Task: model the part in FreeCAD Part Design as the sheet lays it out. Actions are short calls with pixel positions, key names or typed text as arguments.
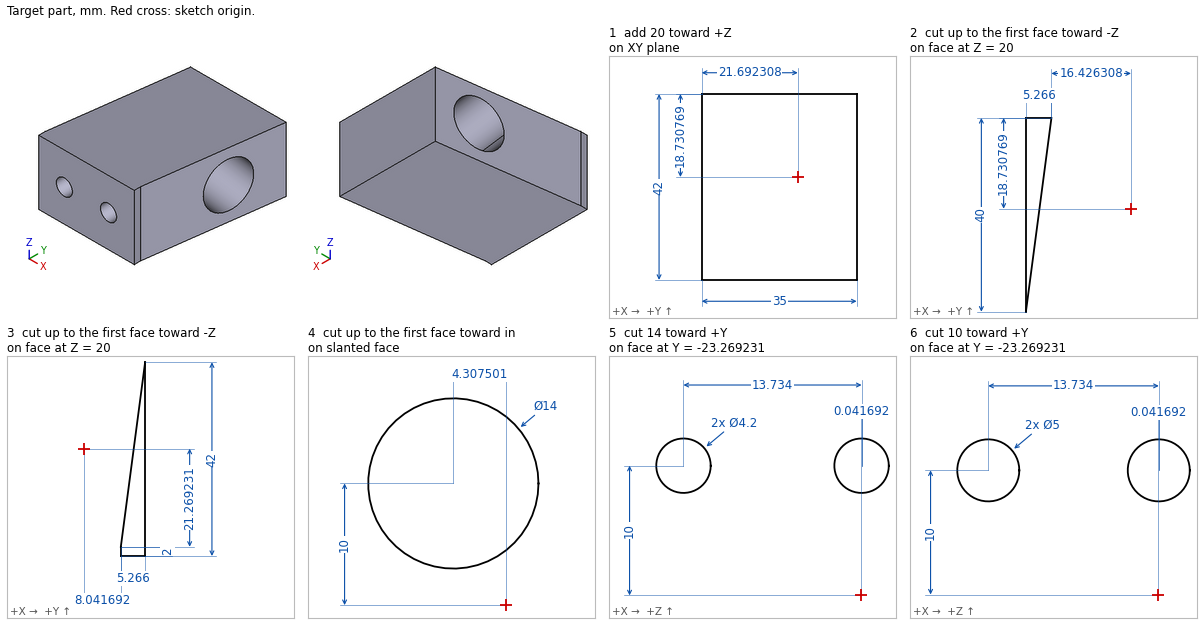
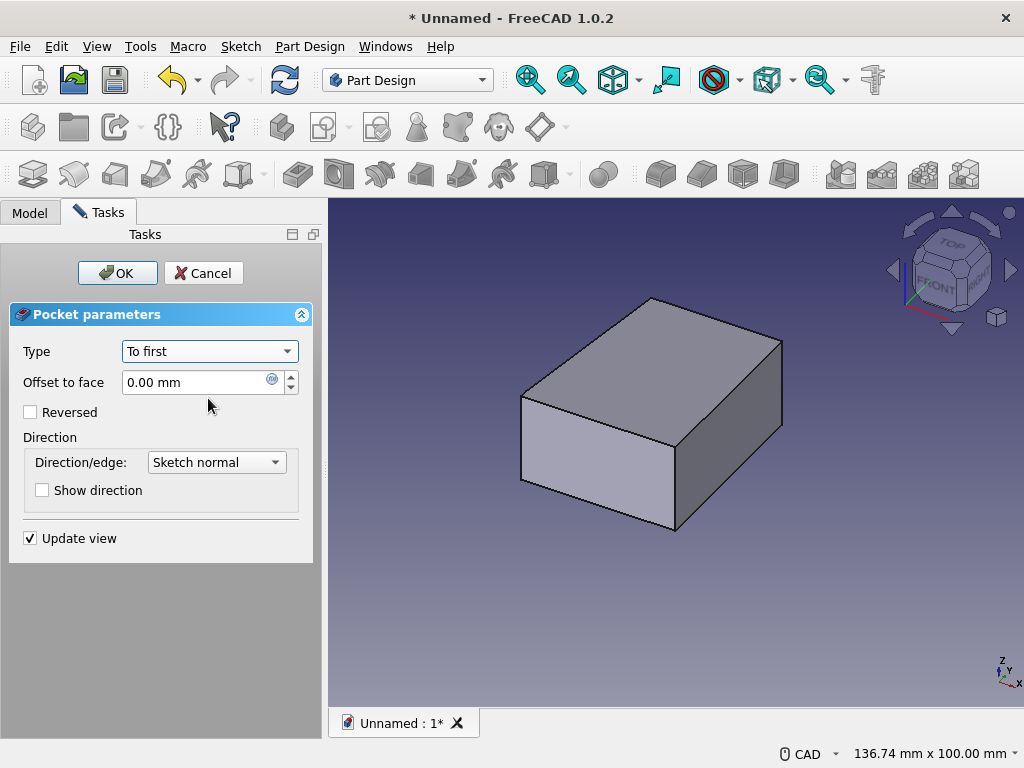
click(118, 273)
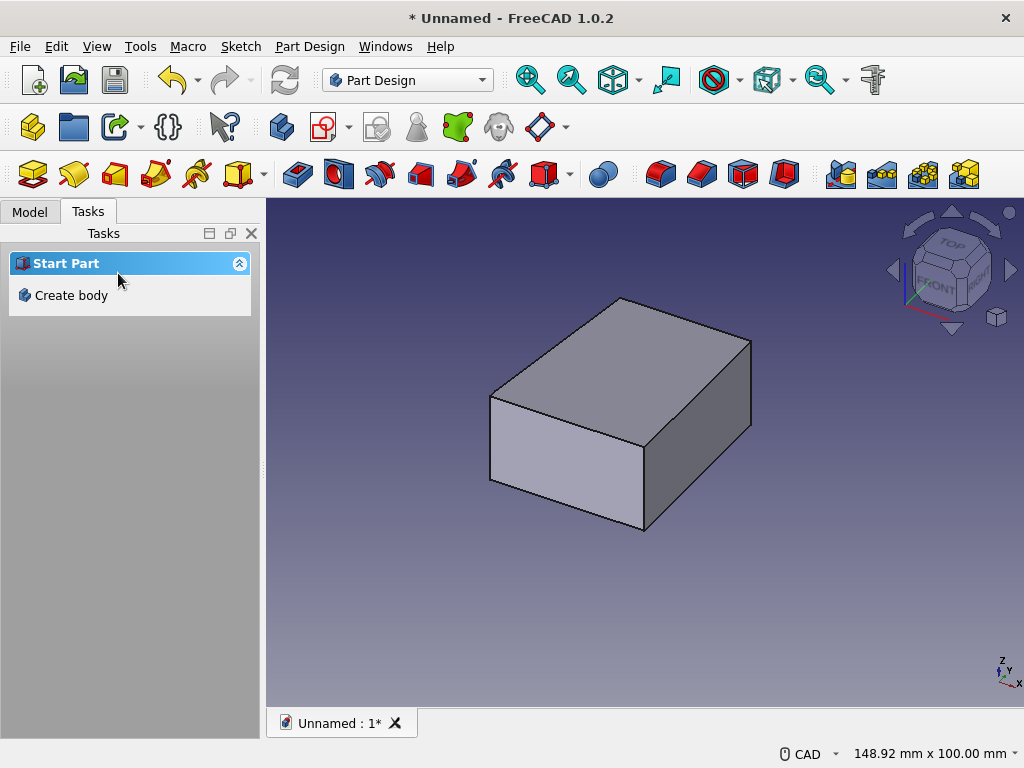
click(605, 383)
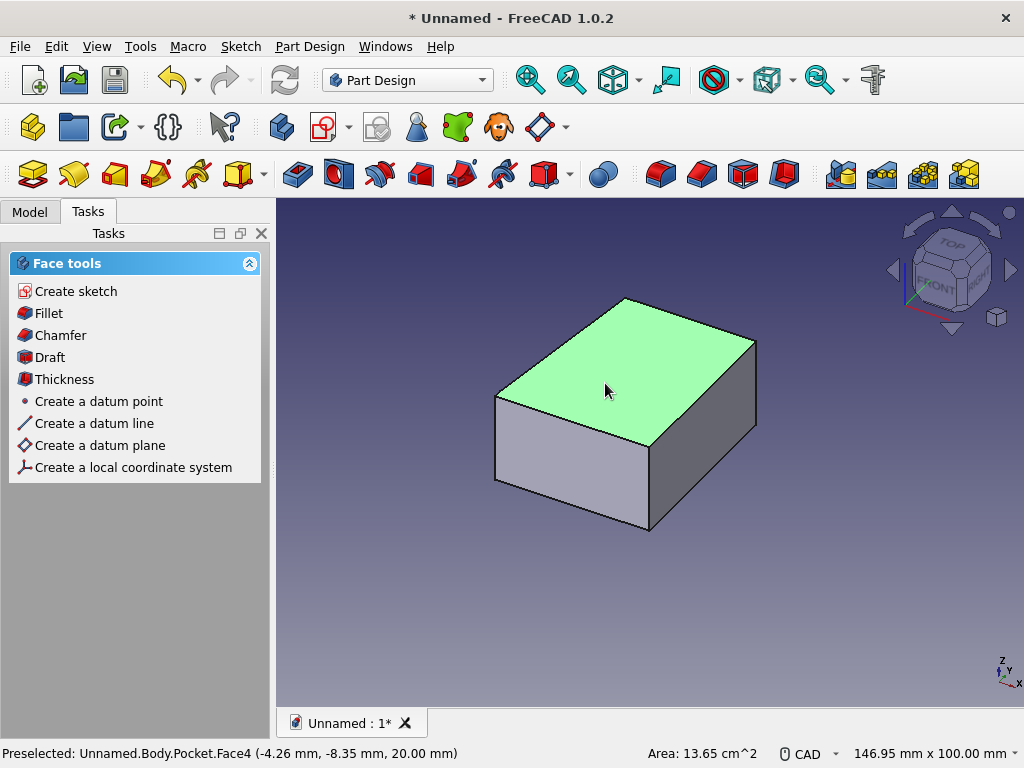
click(322, 128)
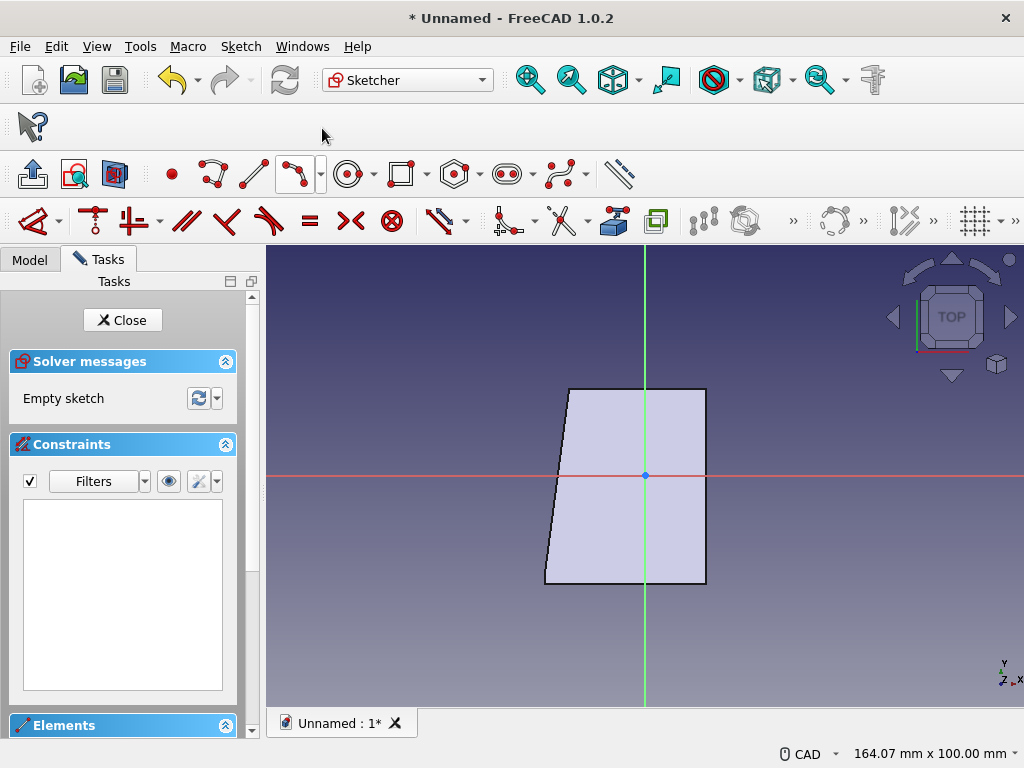
scroll(859, 508, up, 2)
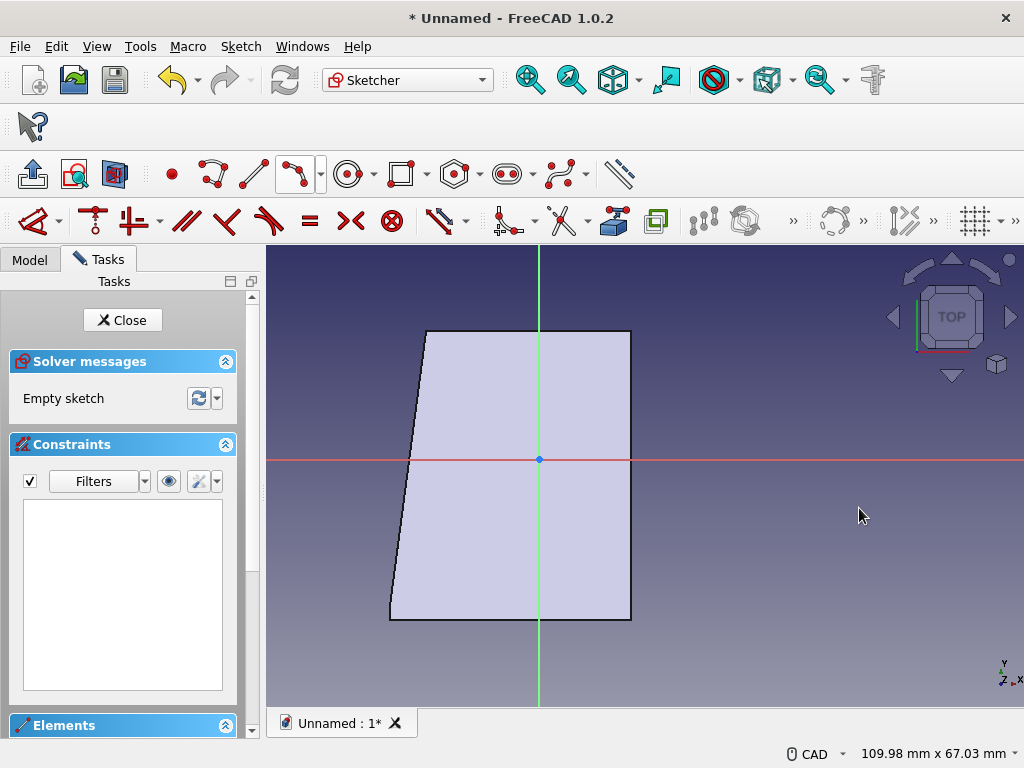
click(213, 174)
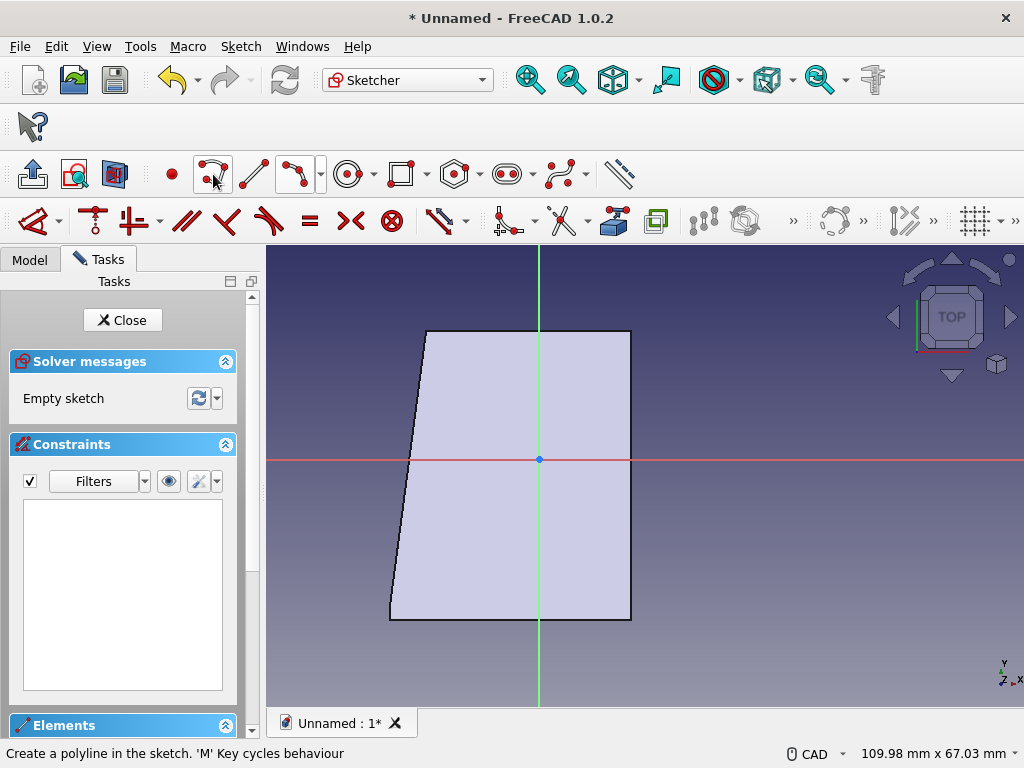
click(595, 607)
click(595, 620)
click(631, 620)
click(631, 331)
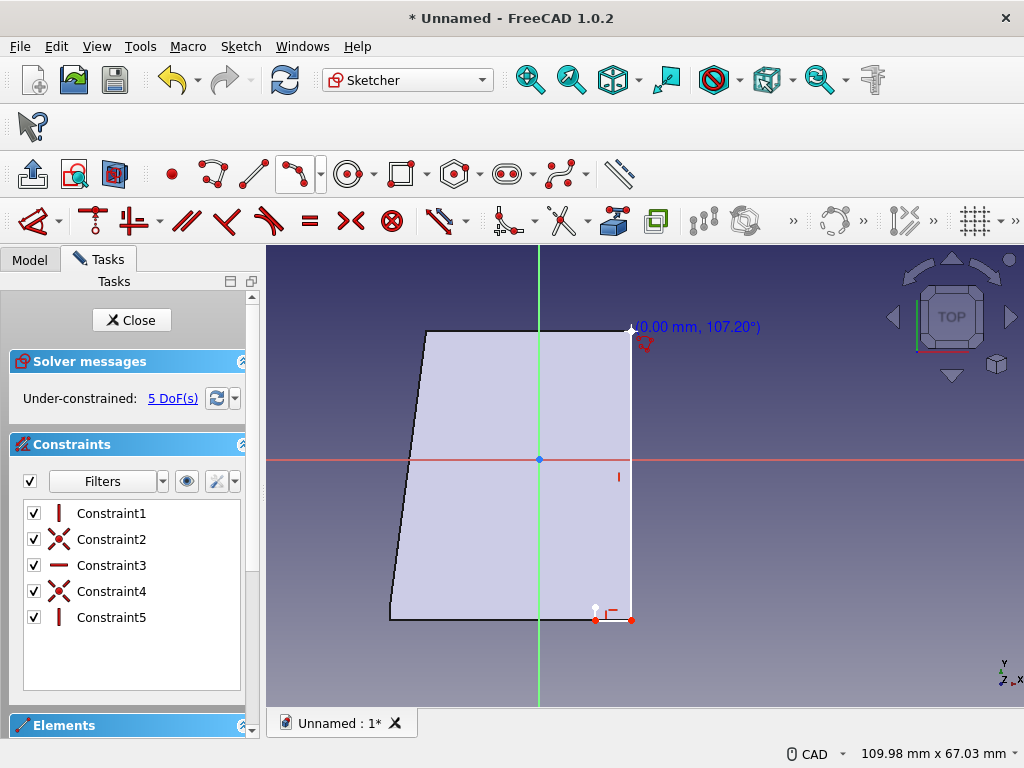
scroll(595, 607, up, 5)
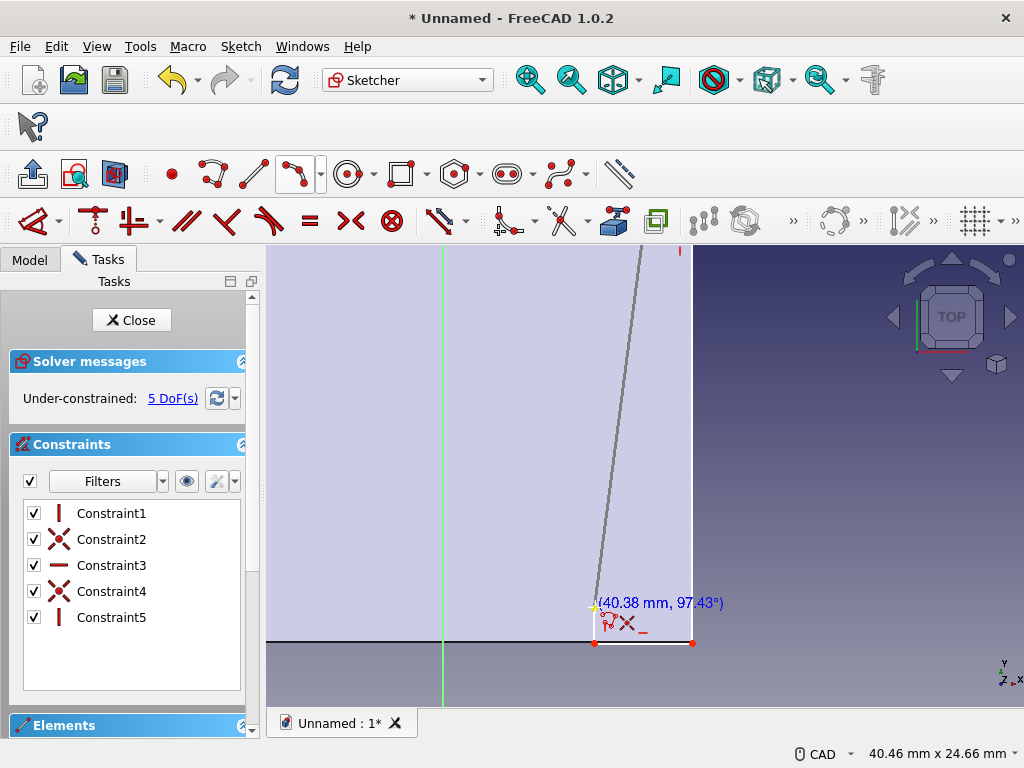
click(594, 608)
key(Escape)
key(Escape)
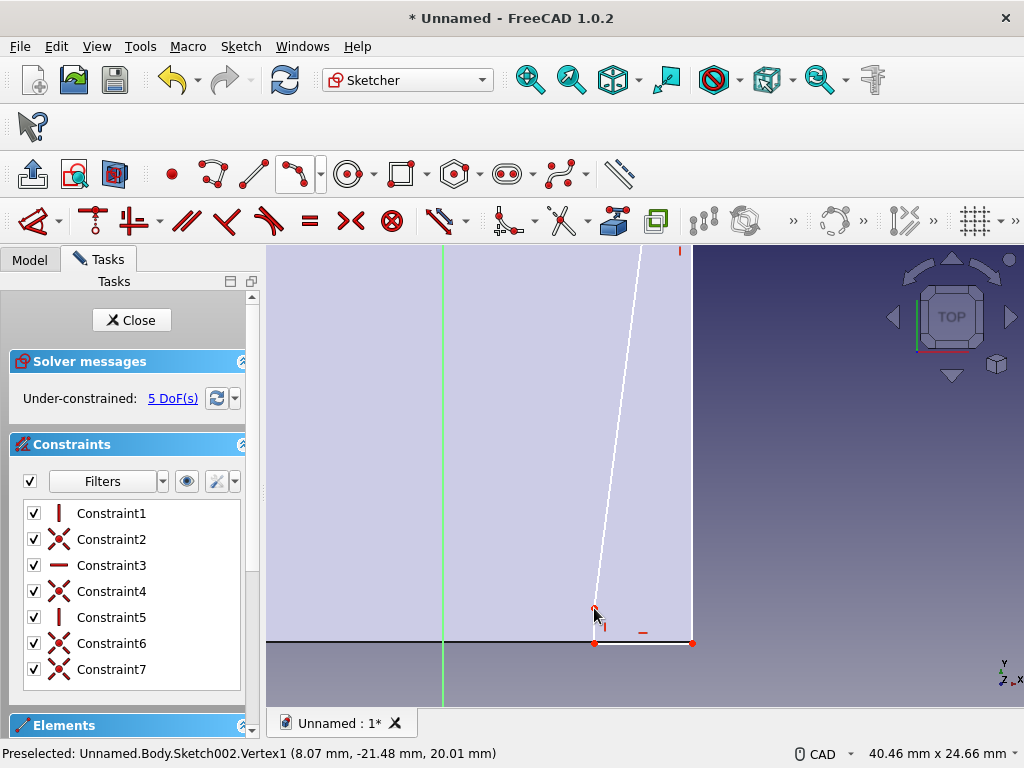
click(32, 222)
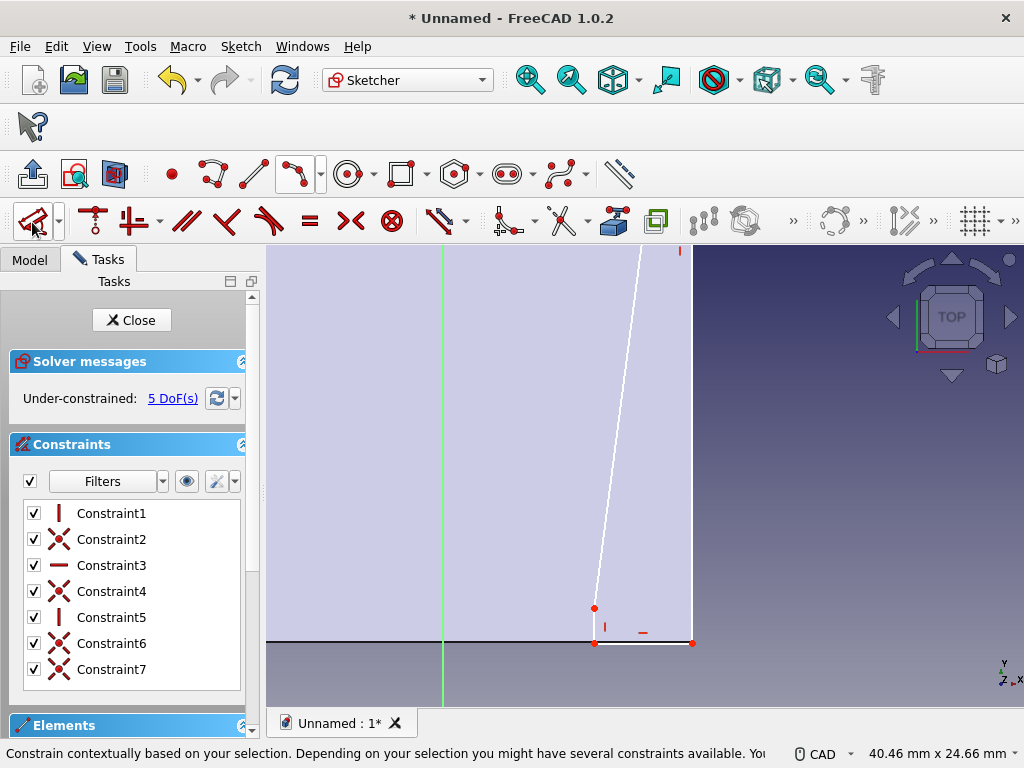
scroll(594, 619, up, 2)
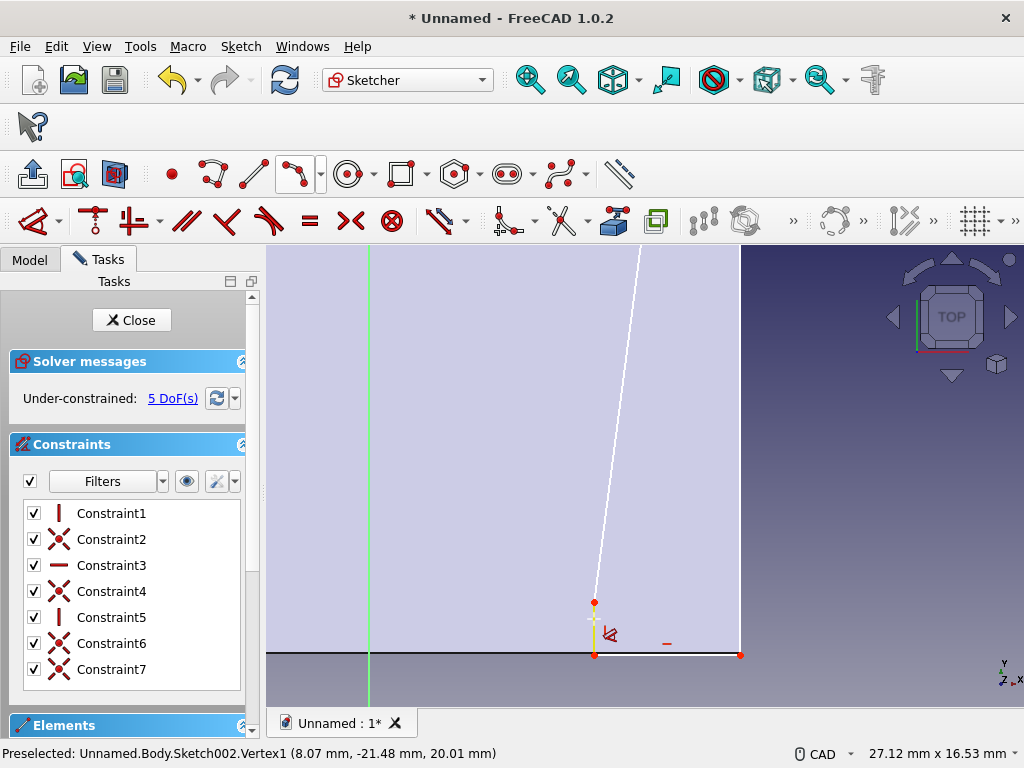
click(594, 619)
click(628, 629)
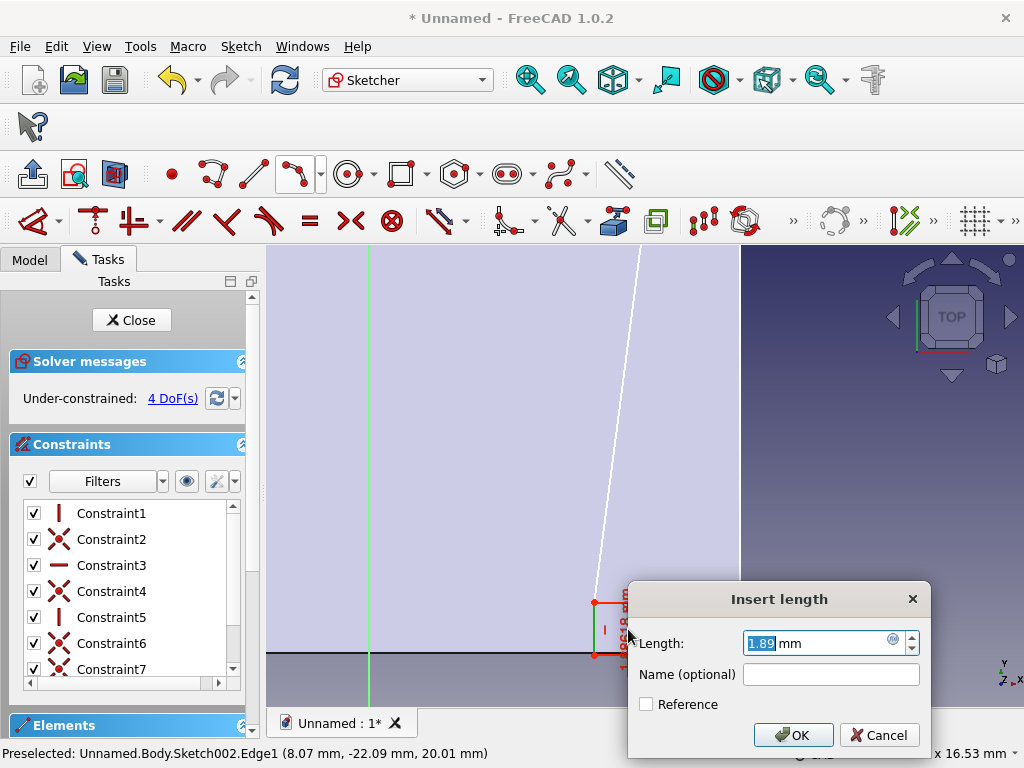
text(2)
key(Return)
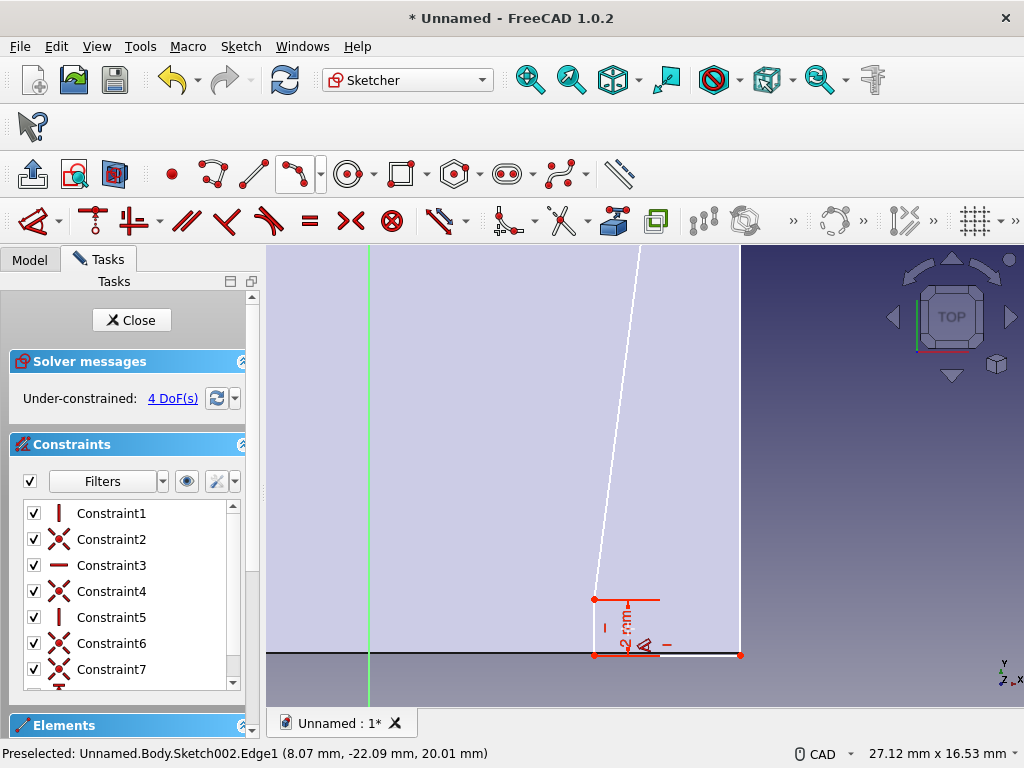
scroll(584, 610, down, 7)